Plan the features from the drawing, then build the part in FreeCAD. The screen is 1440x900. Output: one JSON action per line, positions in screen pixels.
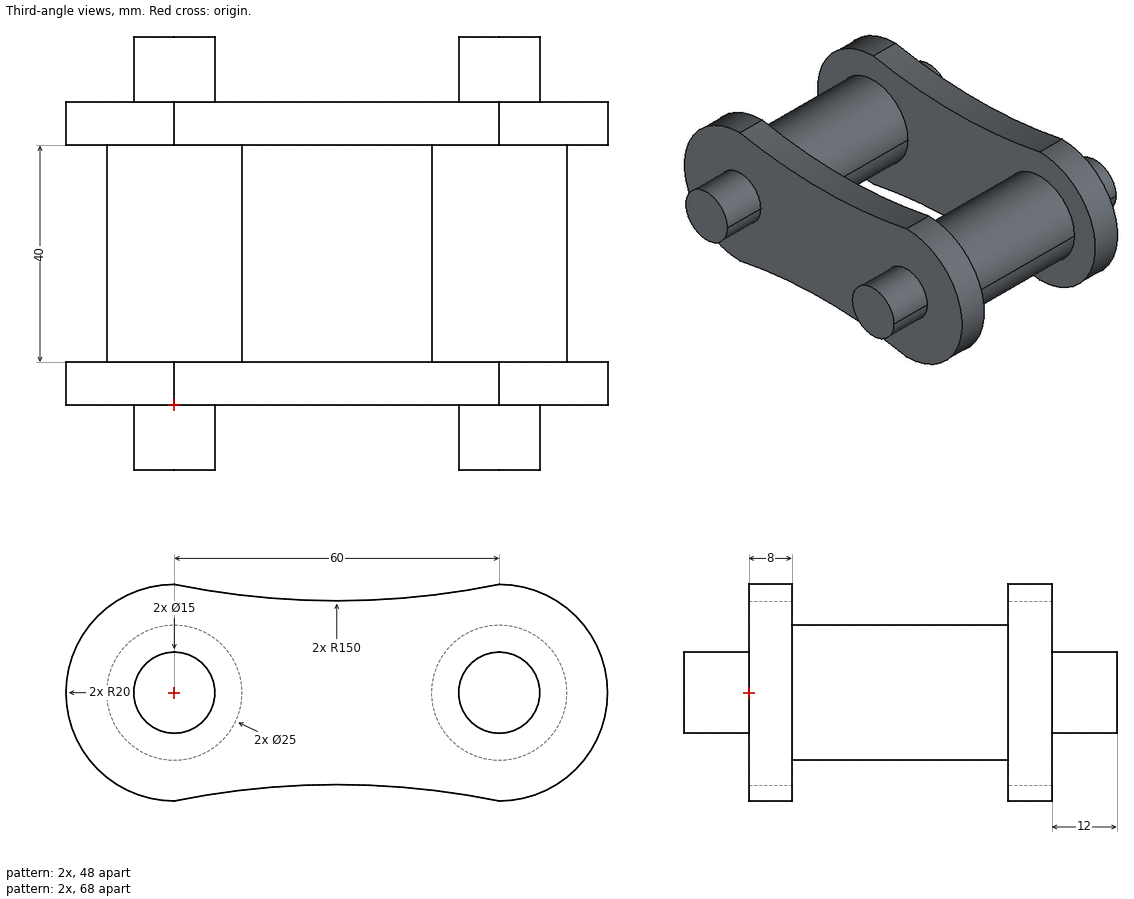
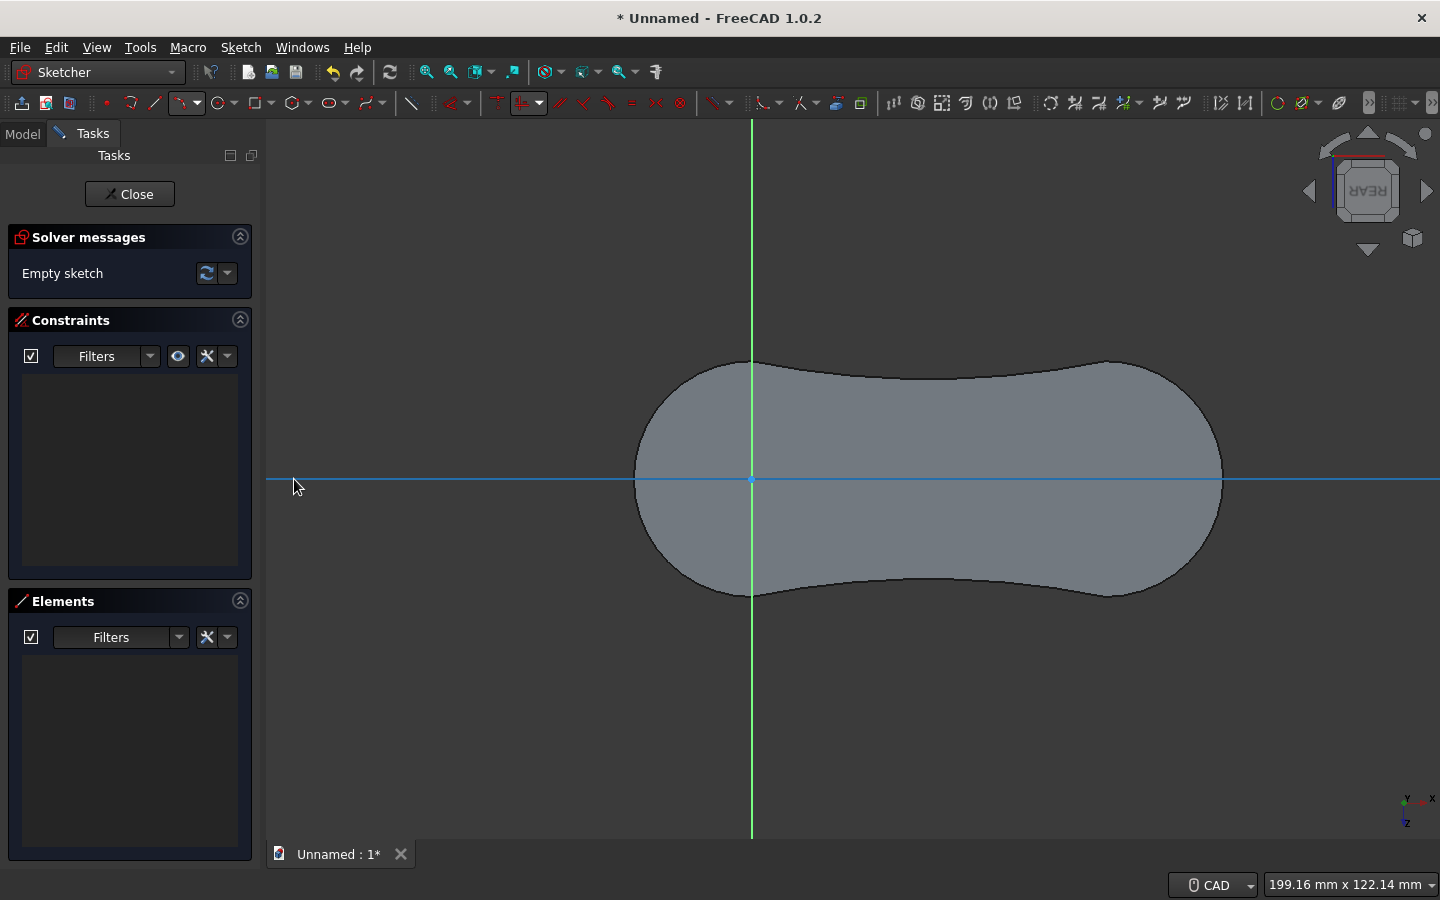
{"action": "scroll", "coordinate": [1221, 479], "scroll_direction": "up", "scroll_amount": 2}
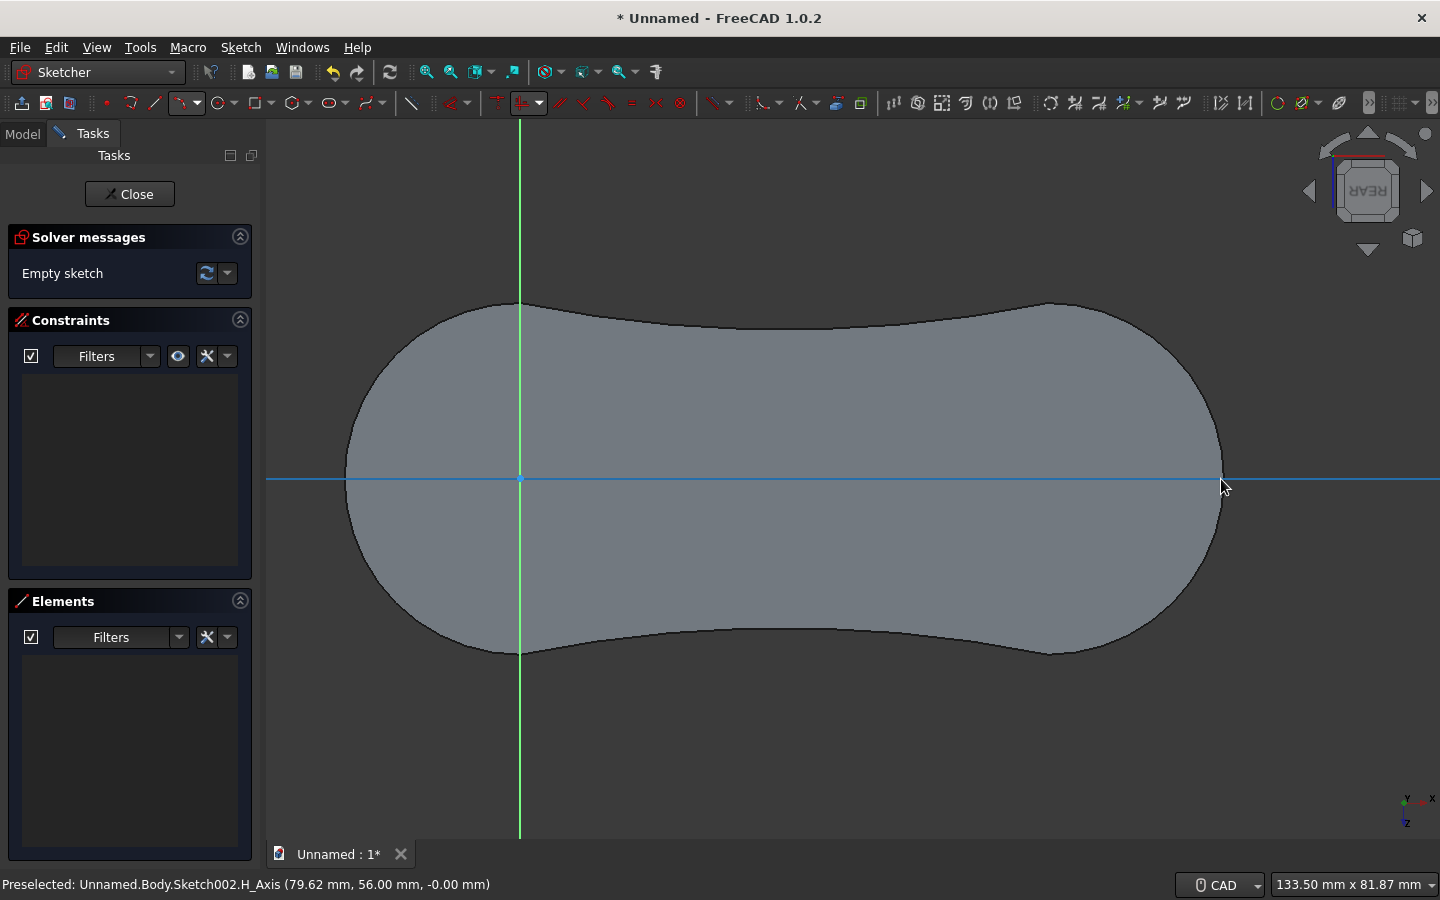
{"action": "left_click", "coordinate": [218, 104]}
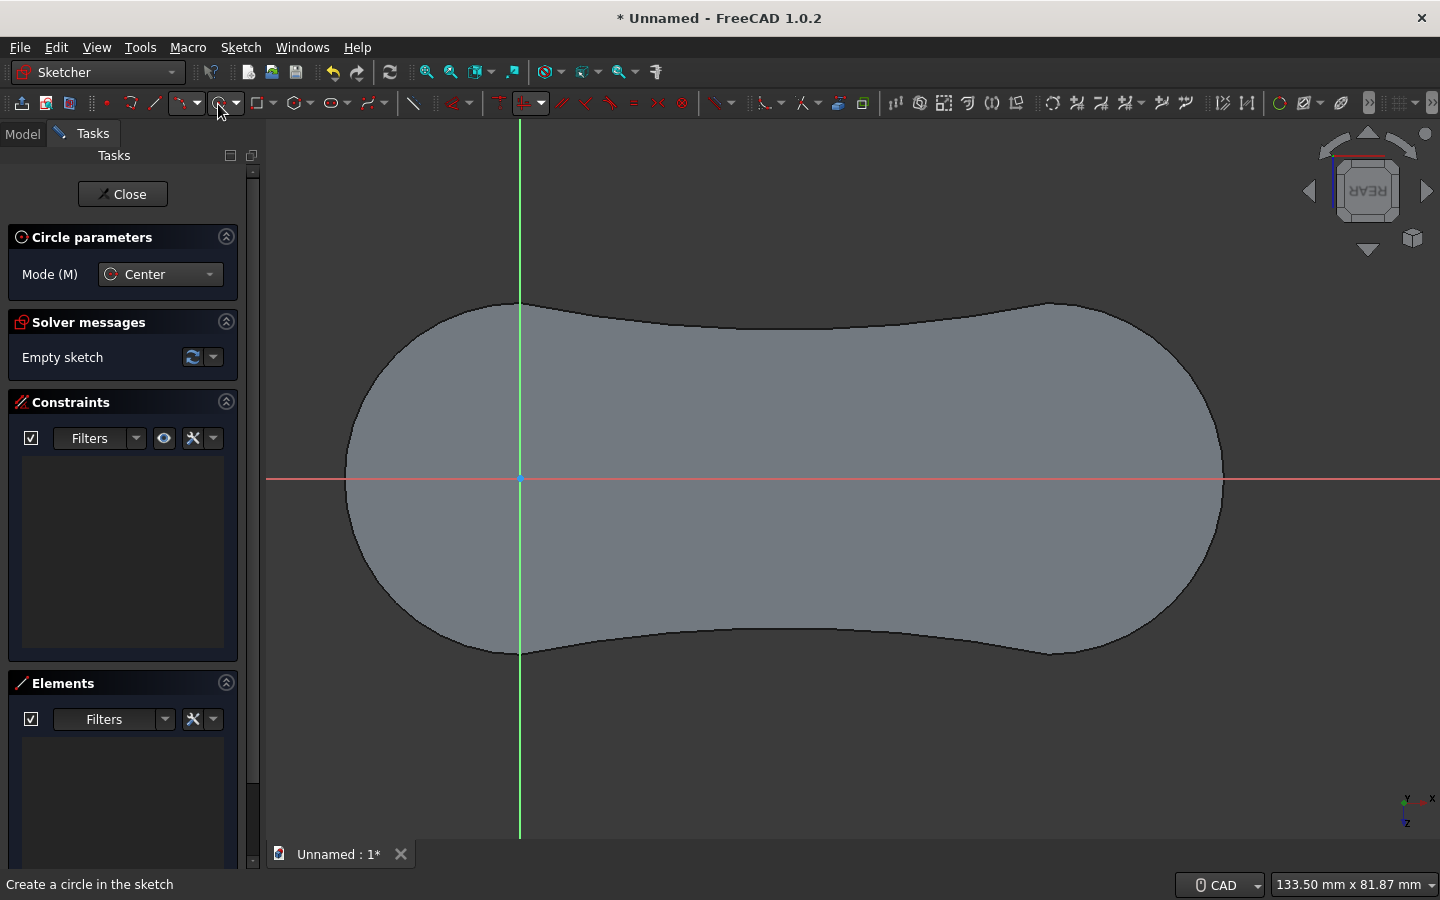
{"action": "left_click", "coordinate": [520, 479]}
{"action": "mouse_move", "coordinate": [567, 432]}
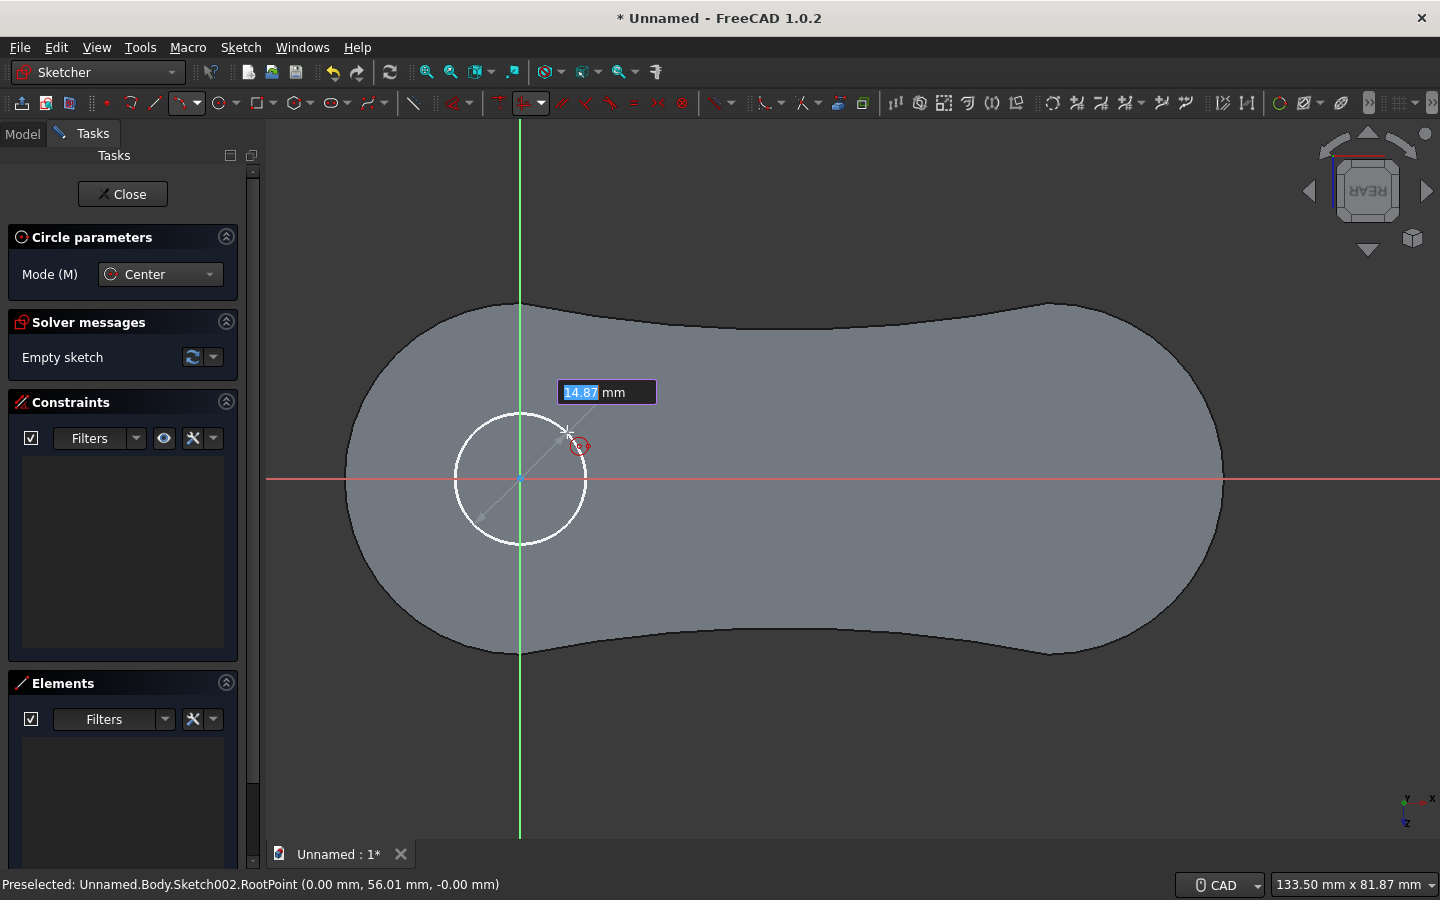
{"action": "type", "text": "15"}
{"action": "key", "text": "Return"}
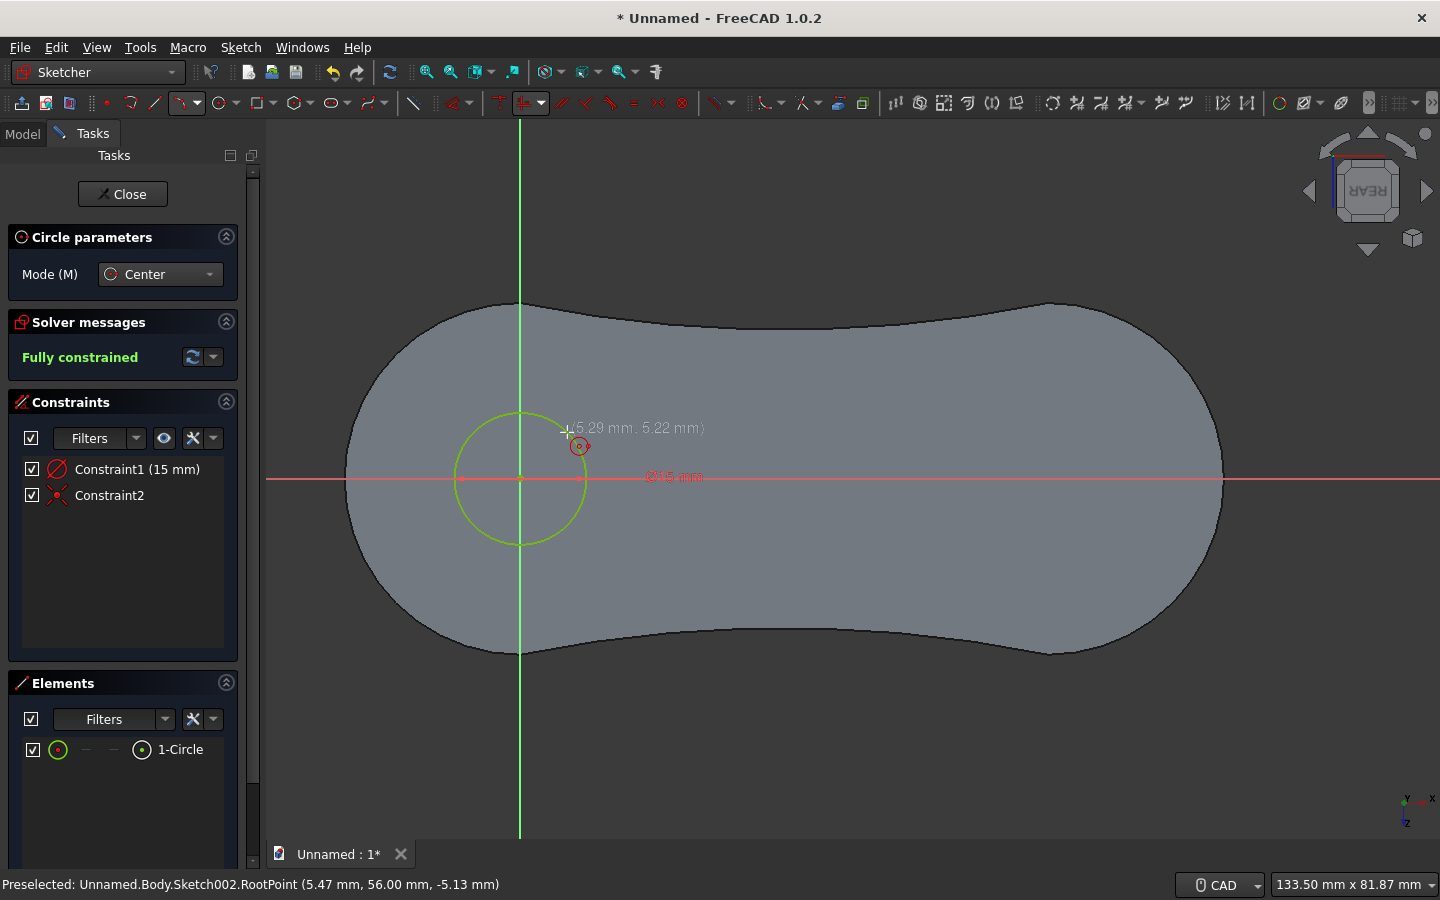
{"action": "left_click", "coordinate": [1048, 479]}
{"action": "mouse_move", "coordinate": [1095, 432]}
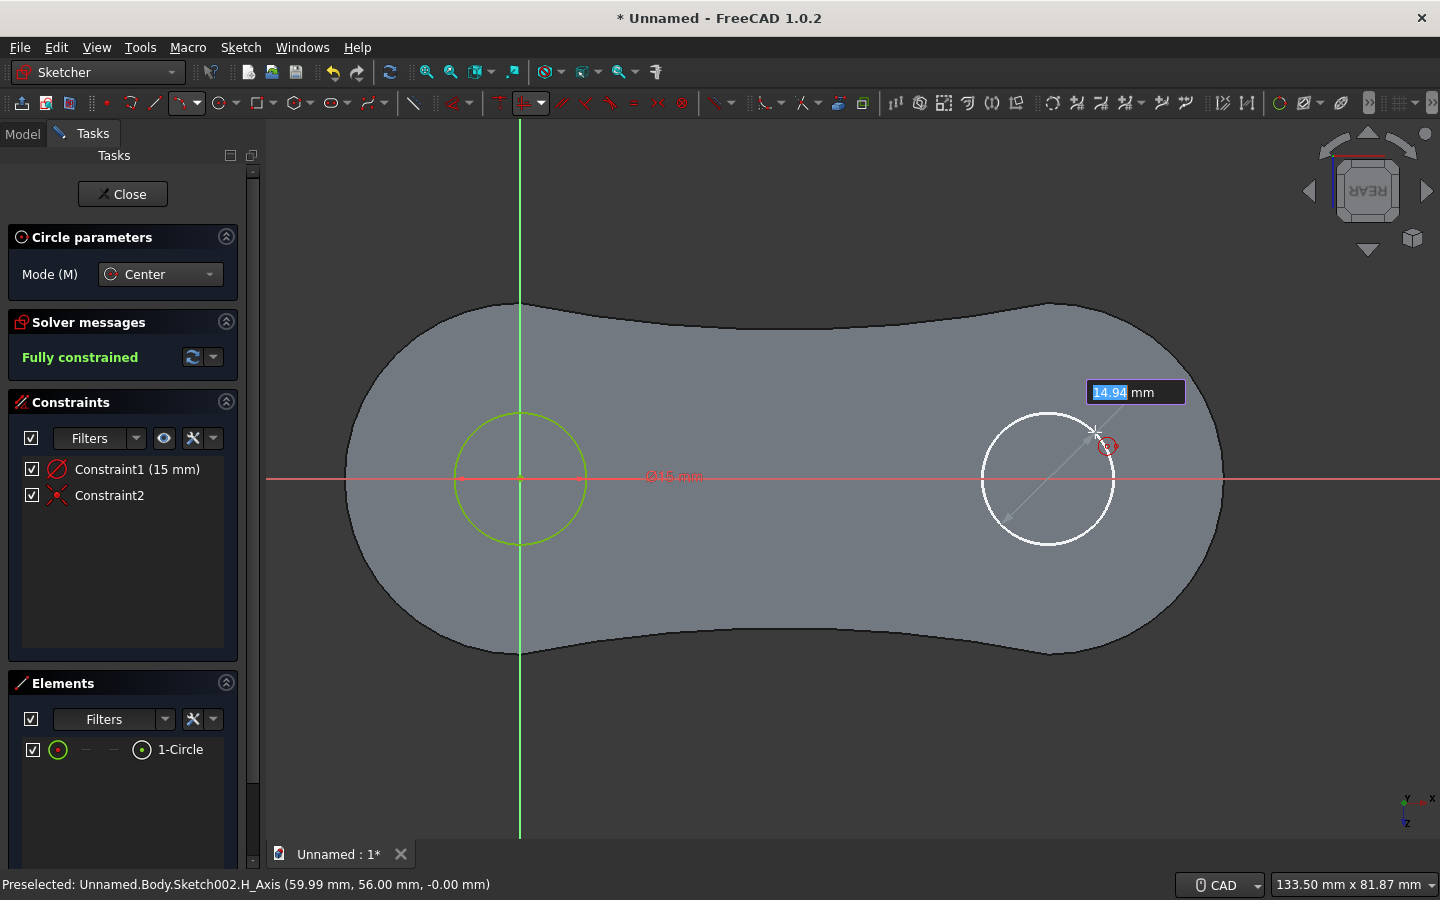
{"action": "type", "text": "15"}
{"action": "key", "text": "Return"}
{"action": "key", "text": "Escape"}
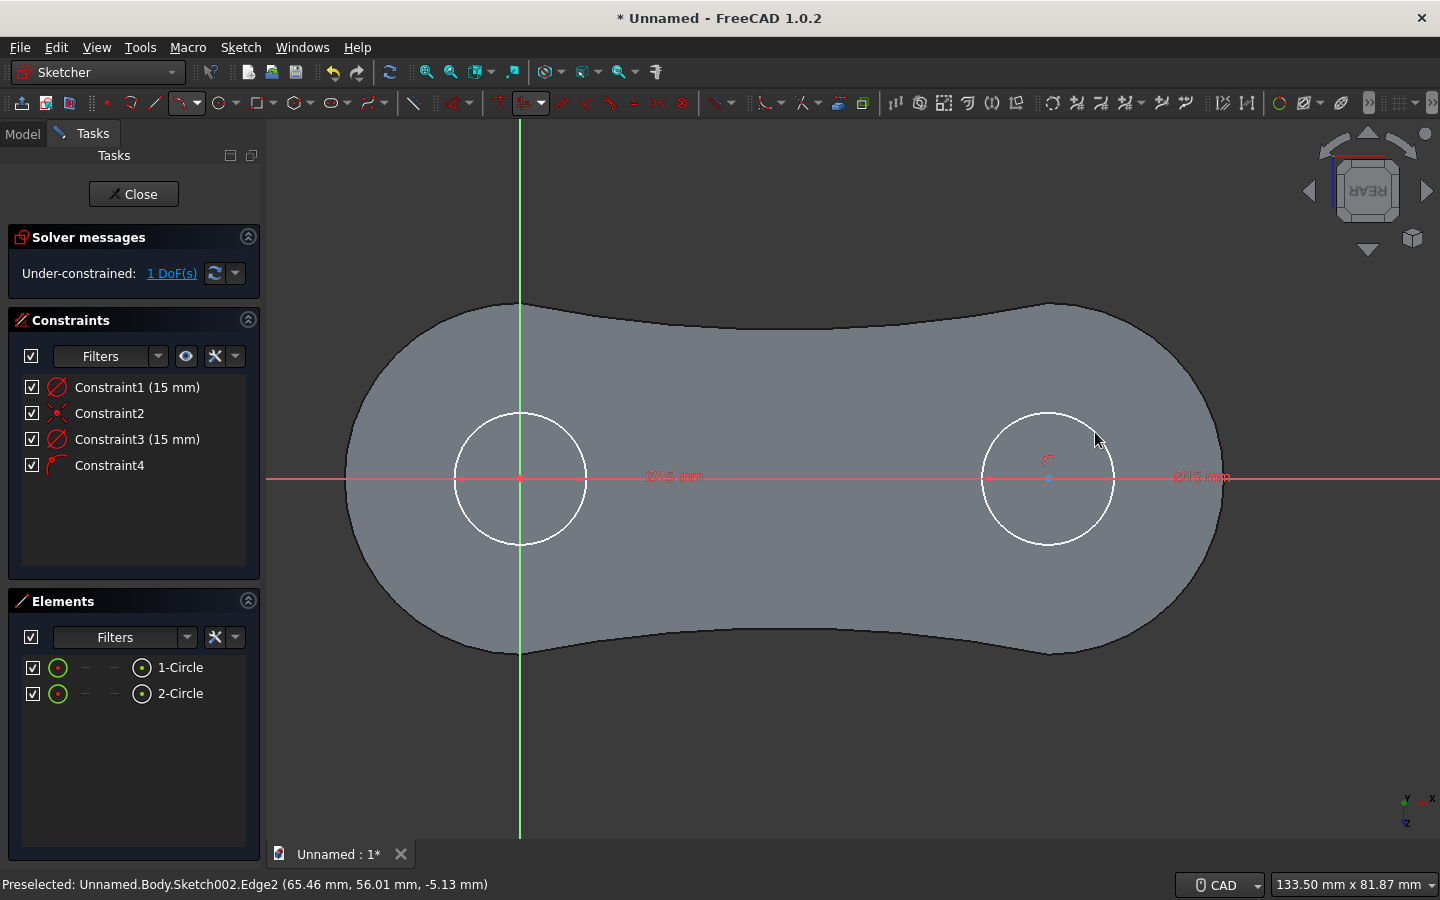
{"action": "left_click", "coordinate": [452, 104]}